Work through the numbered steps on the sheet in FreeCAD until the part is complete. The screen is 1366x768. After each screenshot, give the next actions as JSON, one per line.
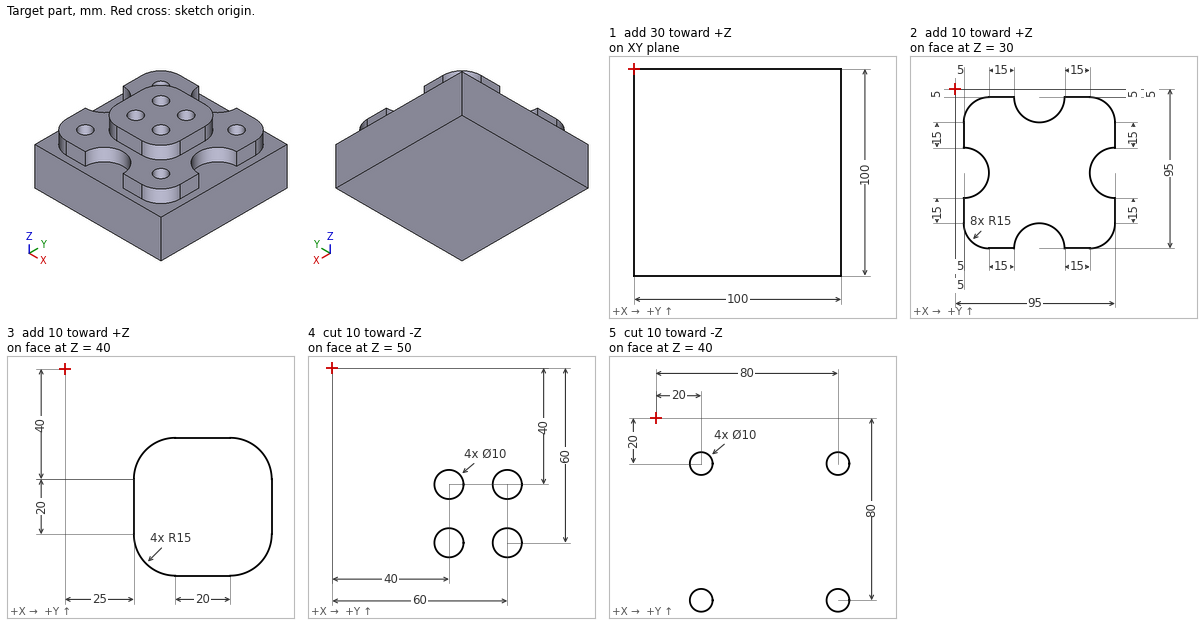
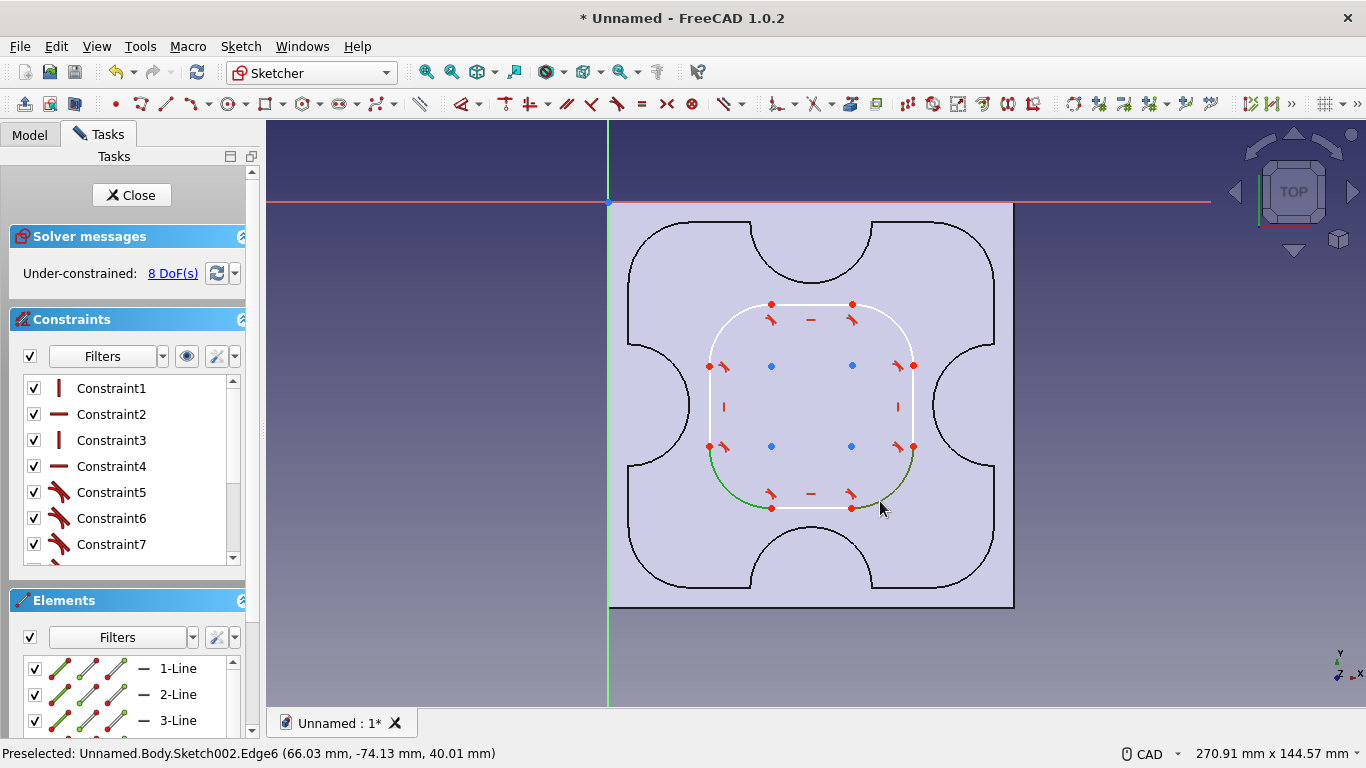
{"action": "left_click", "coordinate": [907, 338]}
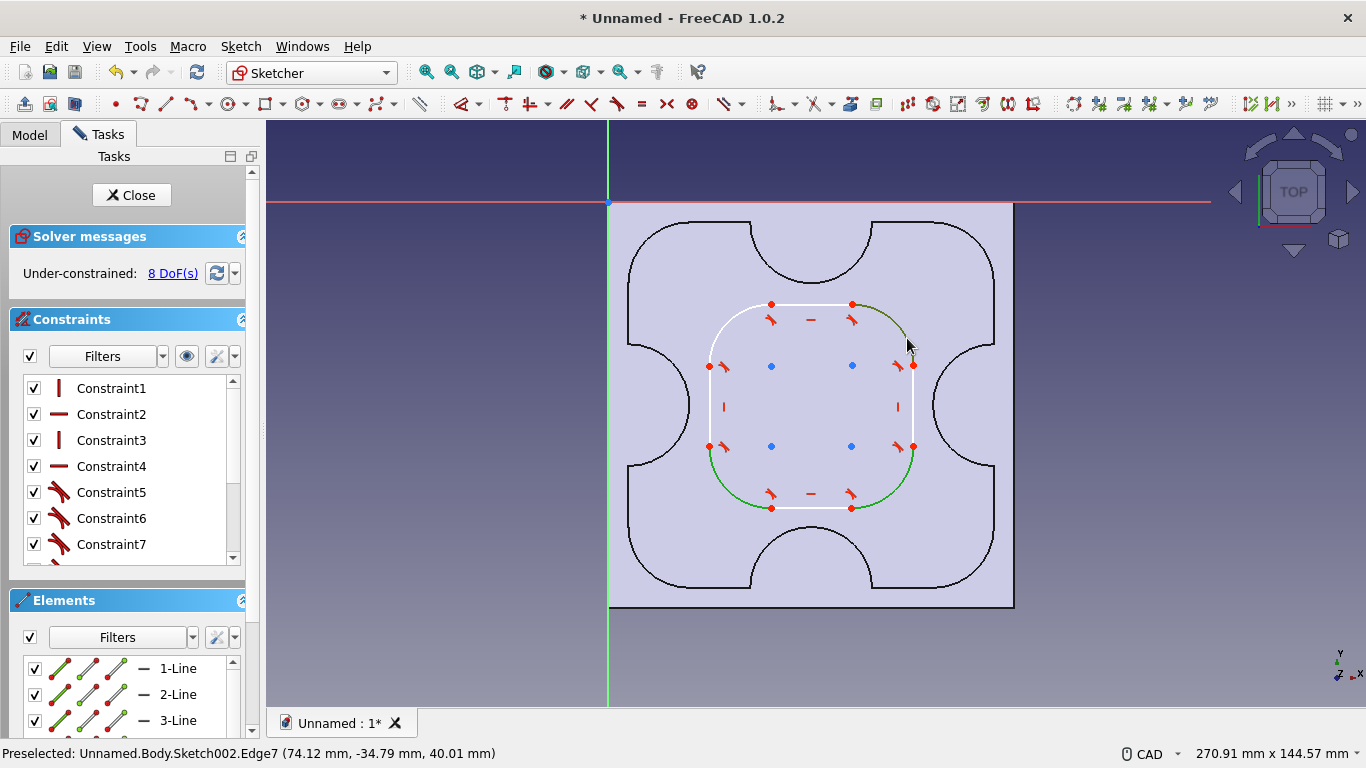
{"action": "left_click", "coordinate": [743, 311]}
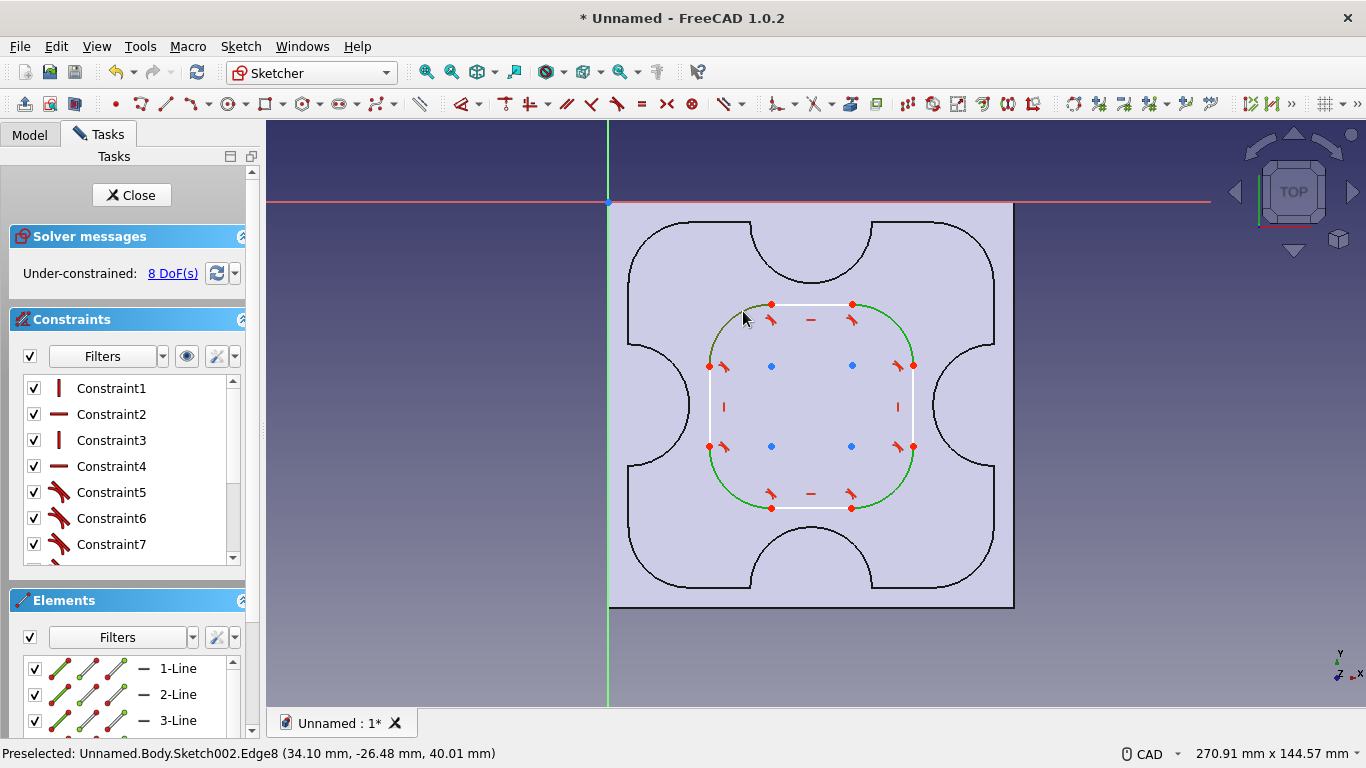
{"action": "left_click", "coordinate": [642, 104]}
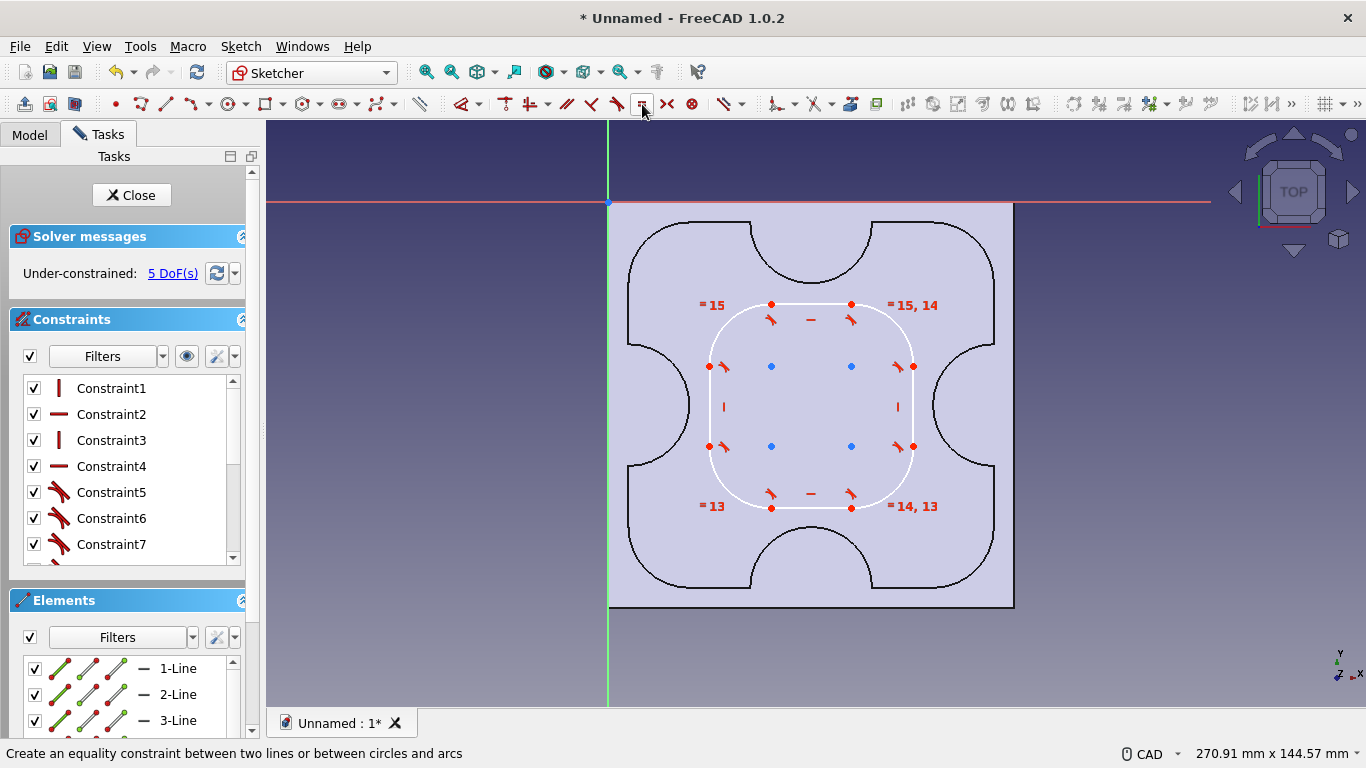
{"action": "left_click", "coordinate": [460, 104]}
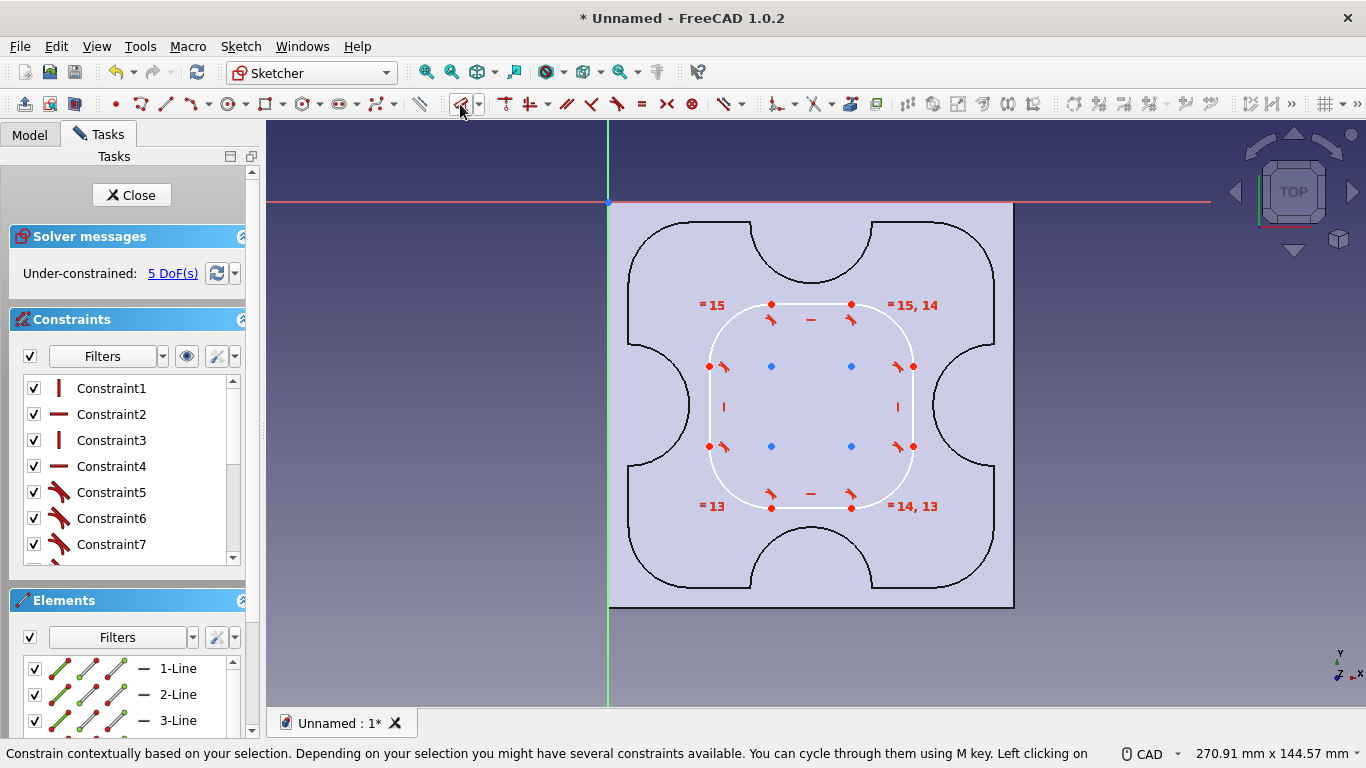
{"action": "left_click", "coordinate": [716, 475]}
{"action": "left_click", "coordinate": [688, 490]}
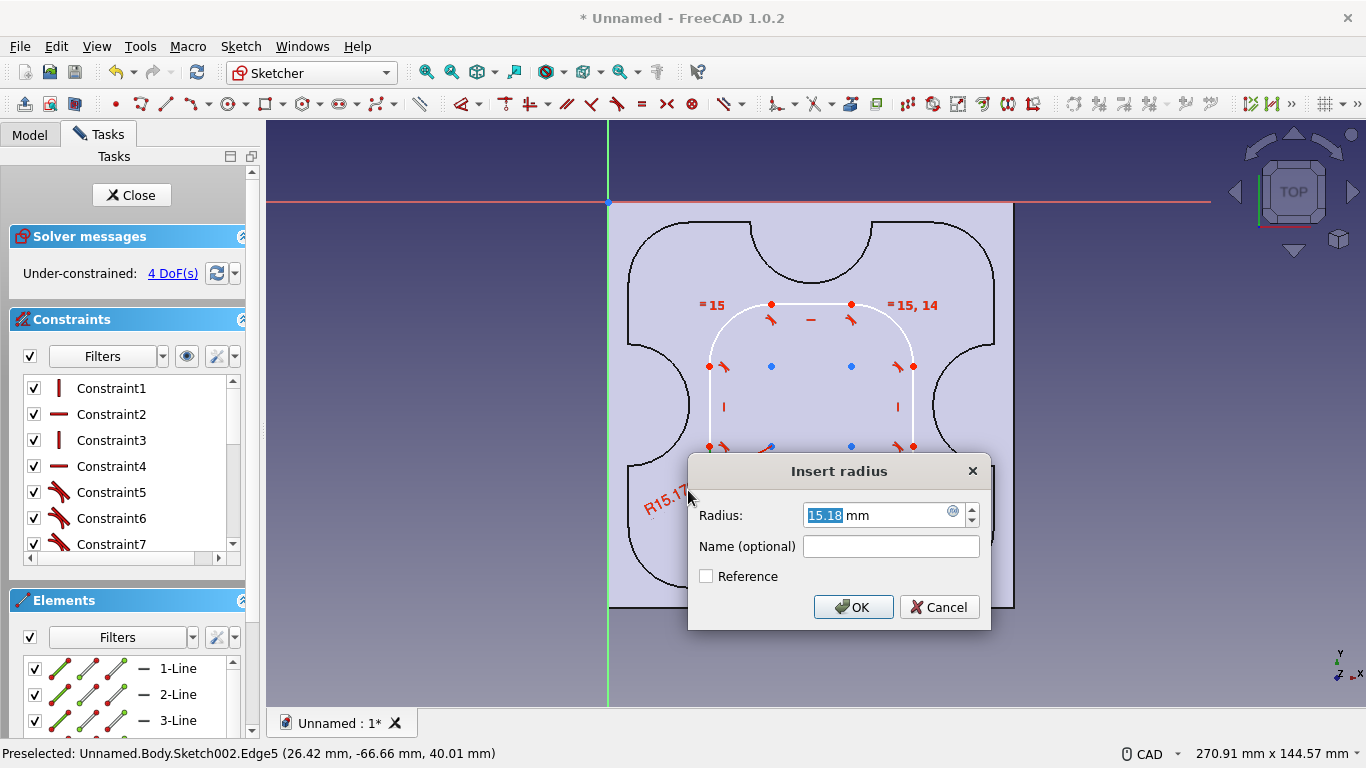
{"action": "type", "text": "15"}
{"action": "key", "text": "Return"}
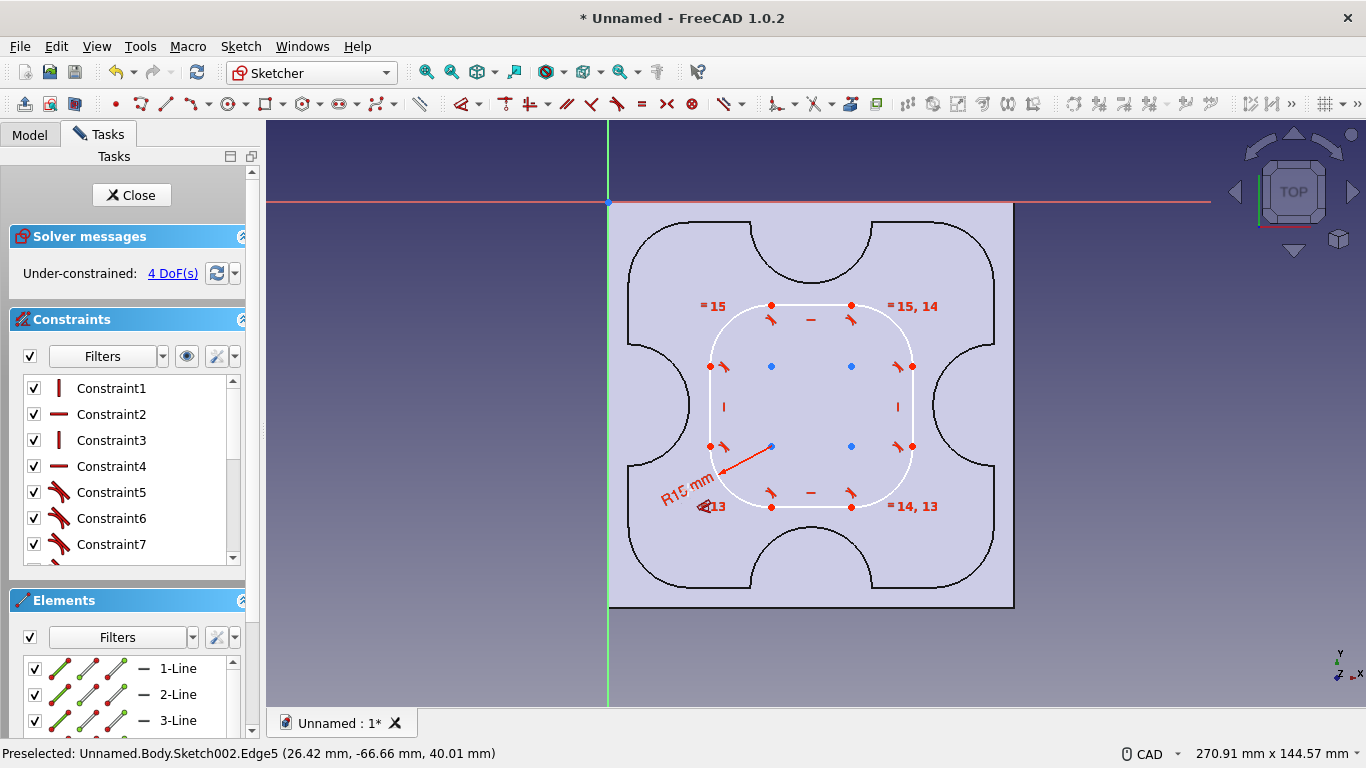
{"action": "left_click", "coordinate": [710, 390]}
{"action": "left_click", "coordinate": [676, 406]}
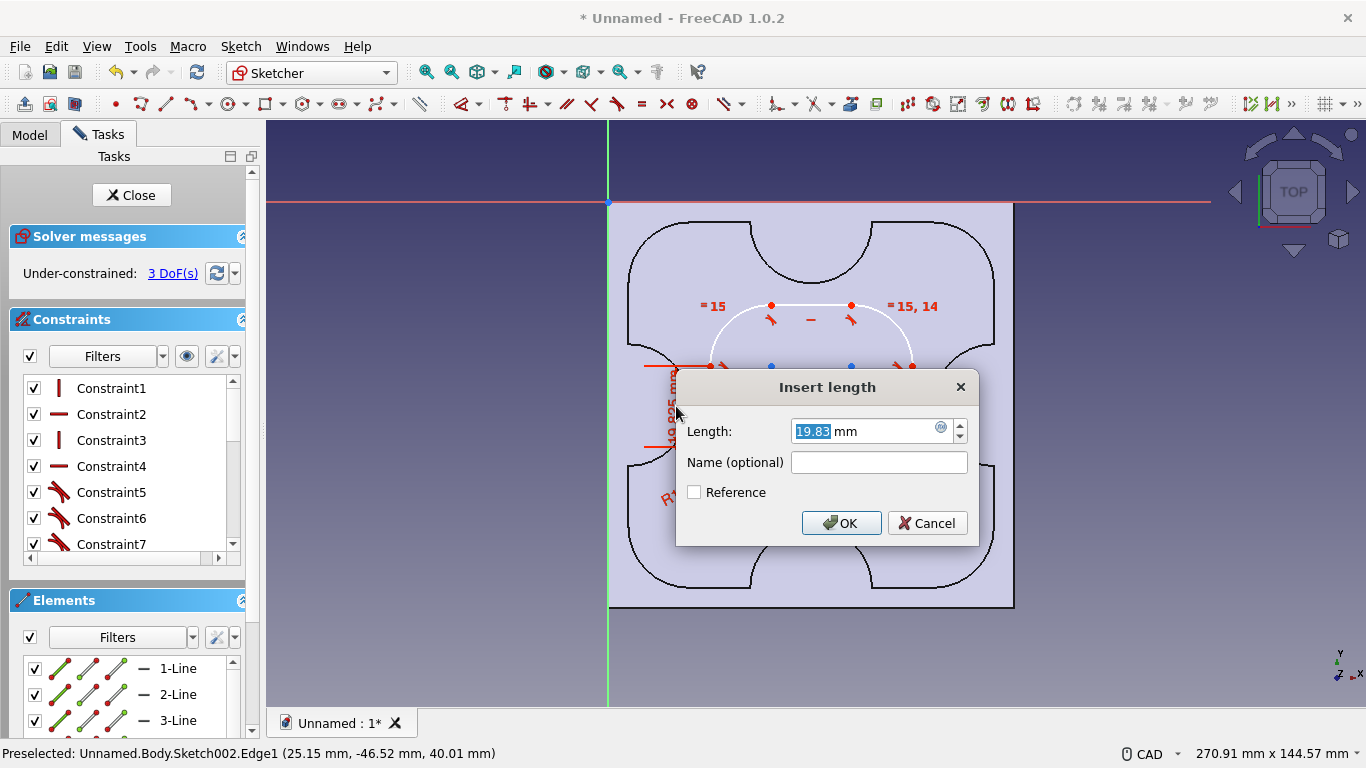
{"action": "type", "text": "20"}
{"action": "key", "text": "Return"}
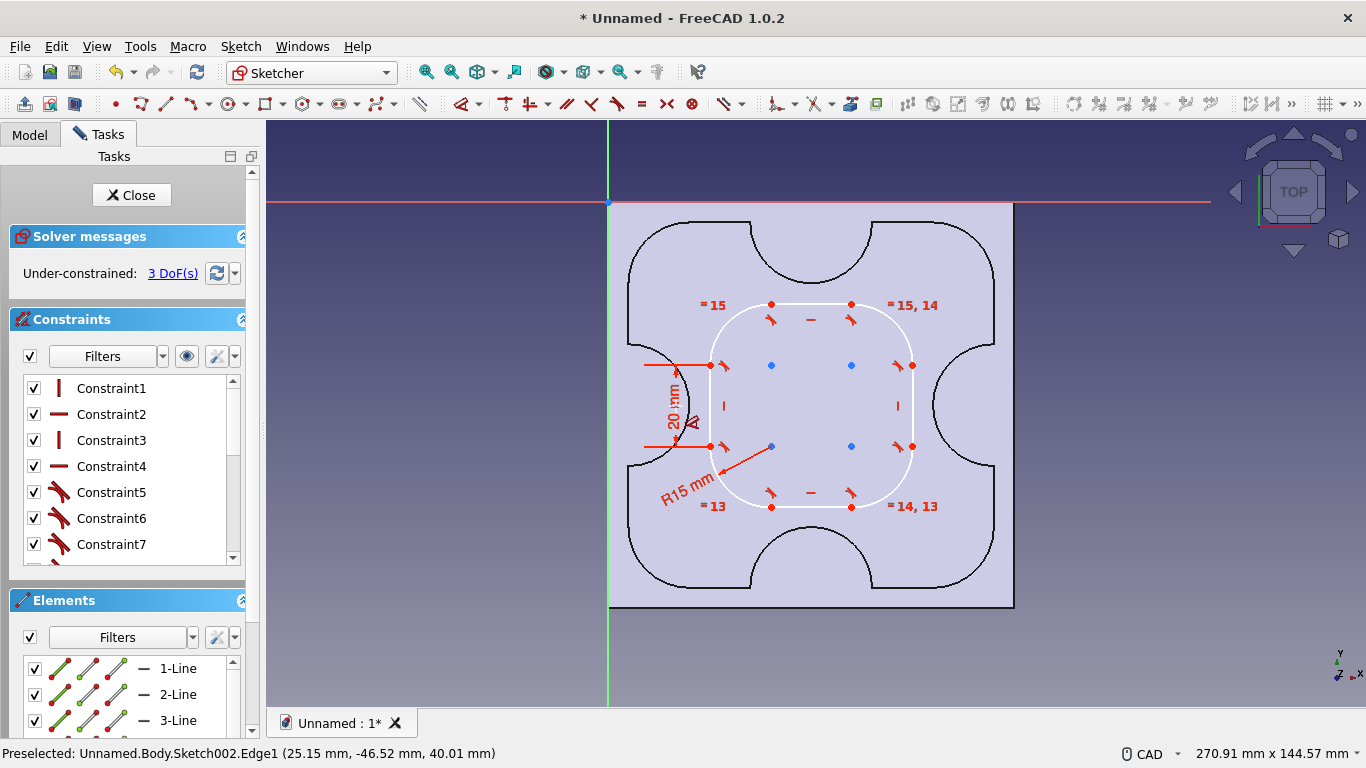
{"action": "left_click", "coordinate": [795, 507]}
{"action": "left_click", "coordinate": [811, 541]}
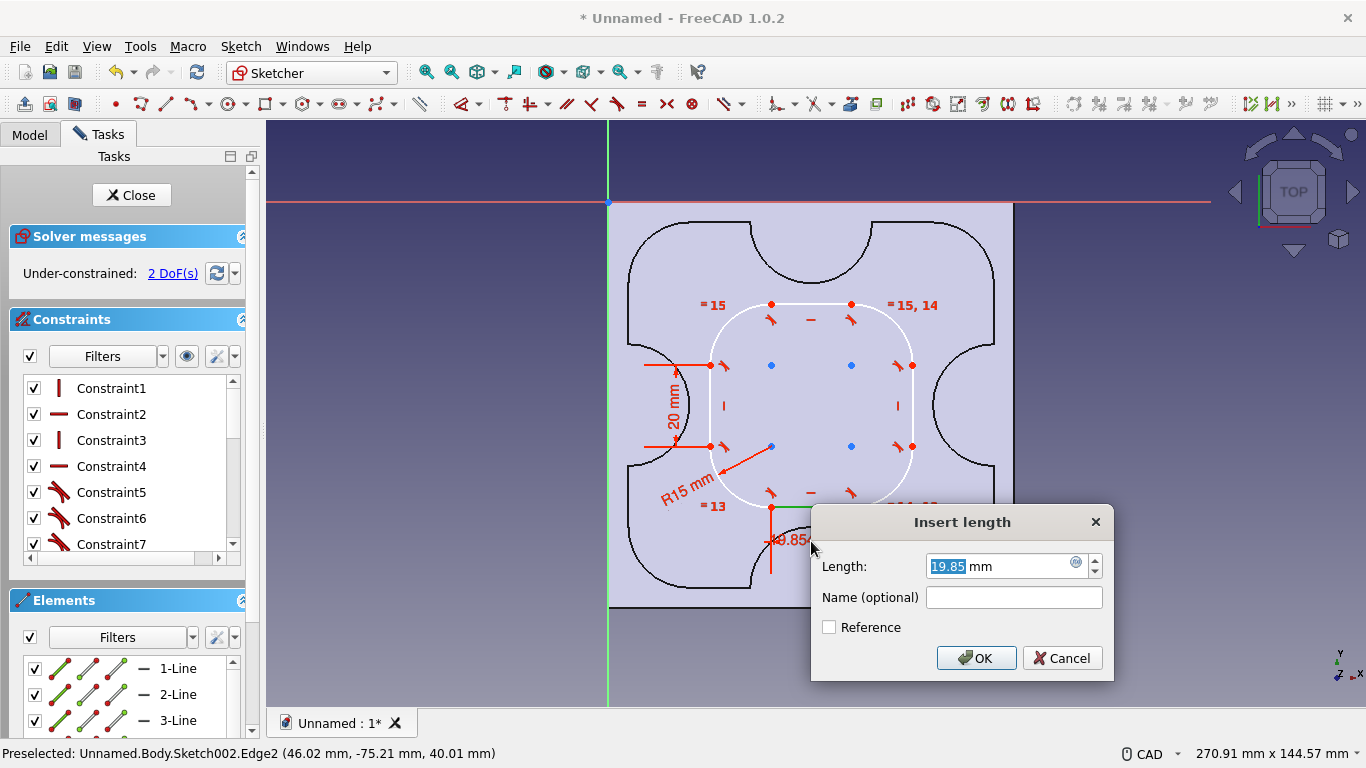
{"action": "type", "text": "20"}
{"action": "key", "text": "Return"}